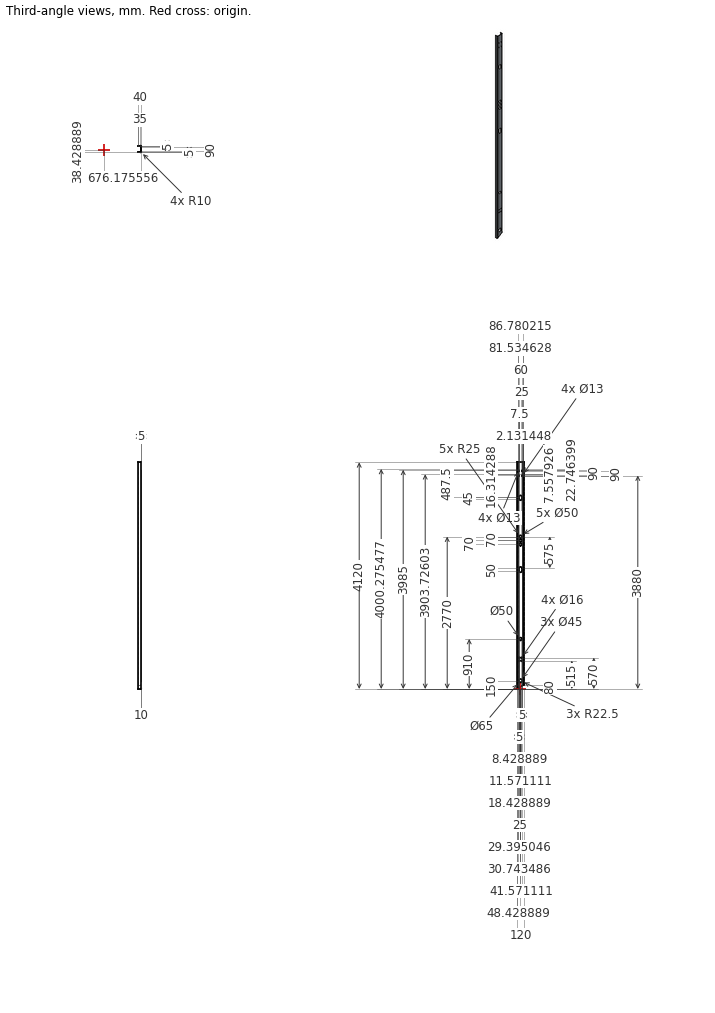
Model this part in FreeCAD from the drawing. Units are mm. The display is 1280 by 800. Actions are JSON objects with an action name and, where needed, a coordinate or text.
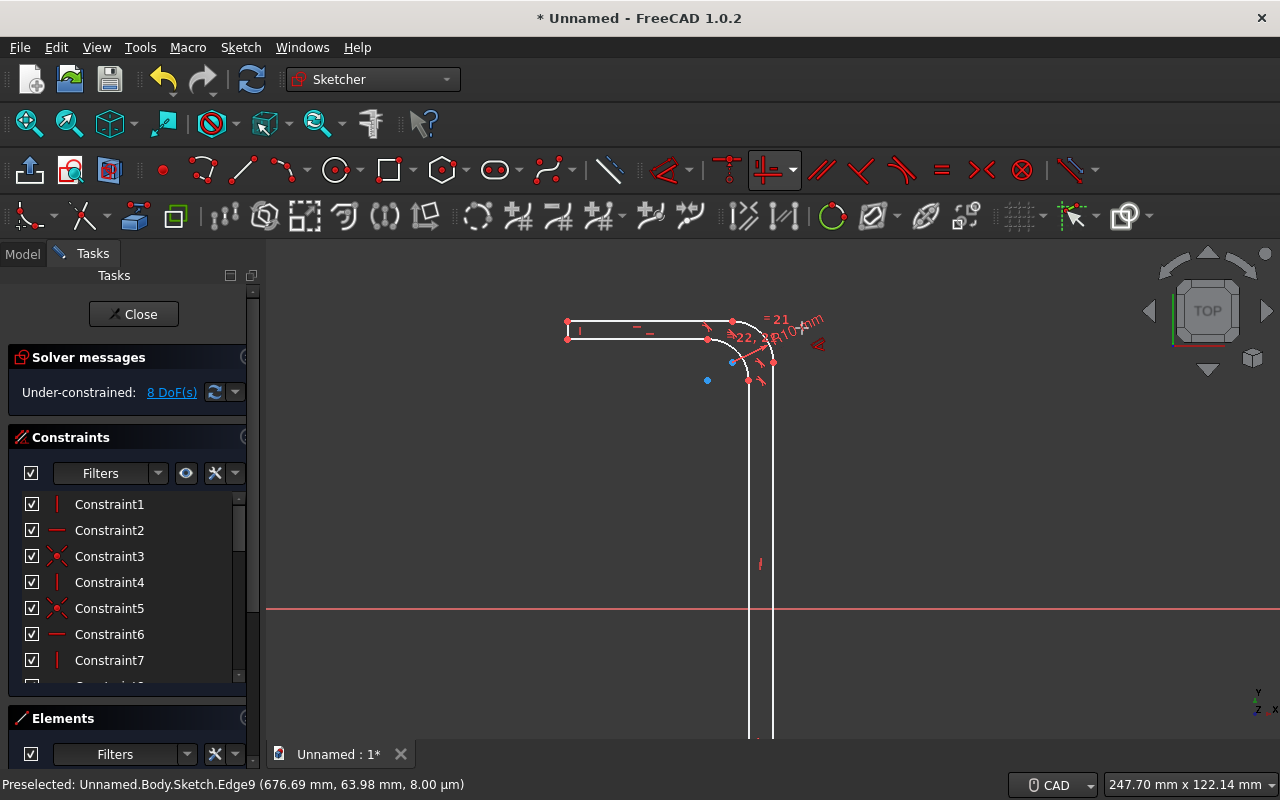
{"action": "scroll", "coordinate": [568, 330], "scroll_direction": "up", "scroll_amount": 4}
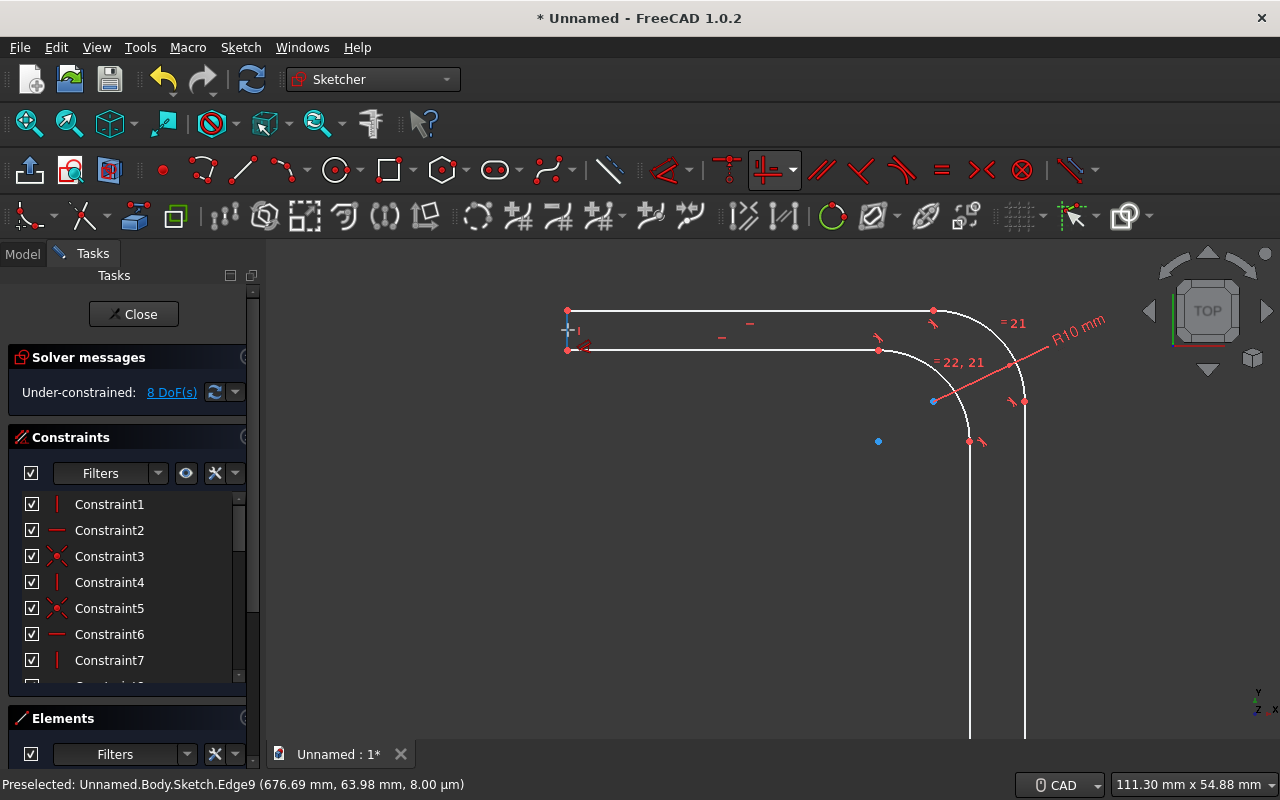
{"action": "left_click", "coordinate": [567, 330]}
{"action": "left_click", "coordinate": [533, 330]}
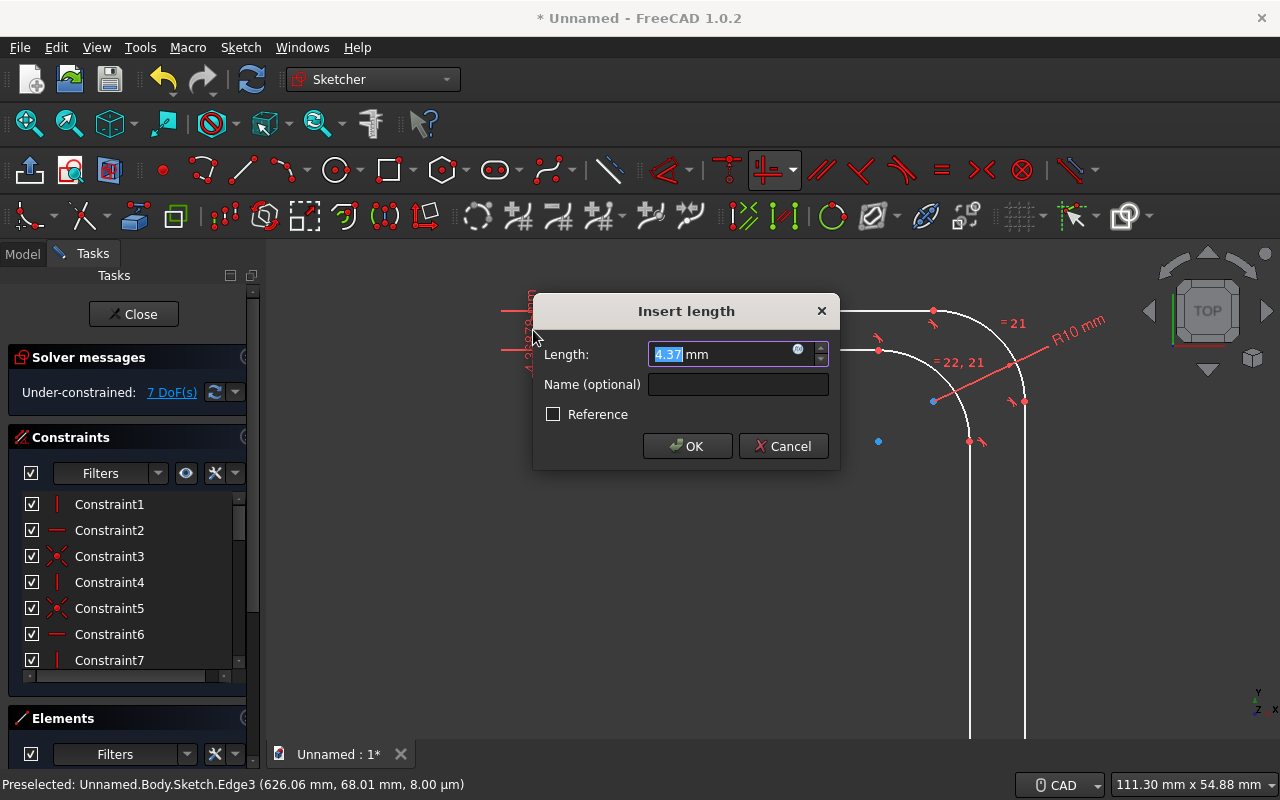
{"action": "type", "text": "5"}
{"action": "key", "text": "Return"}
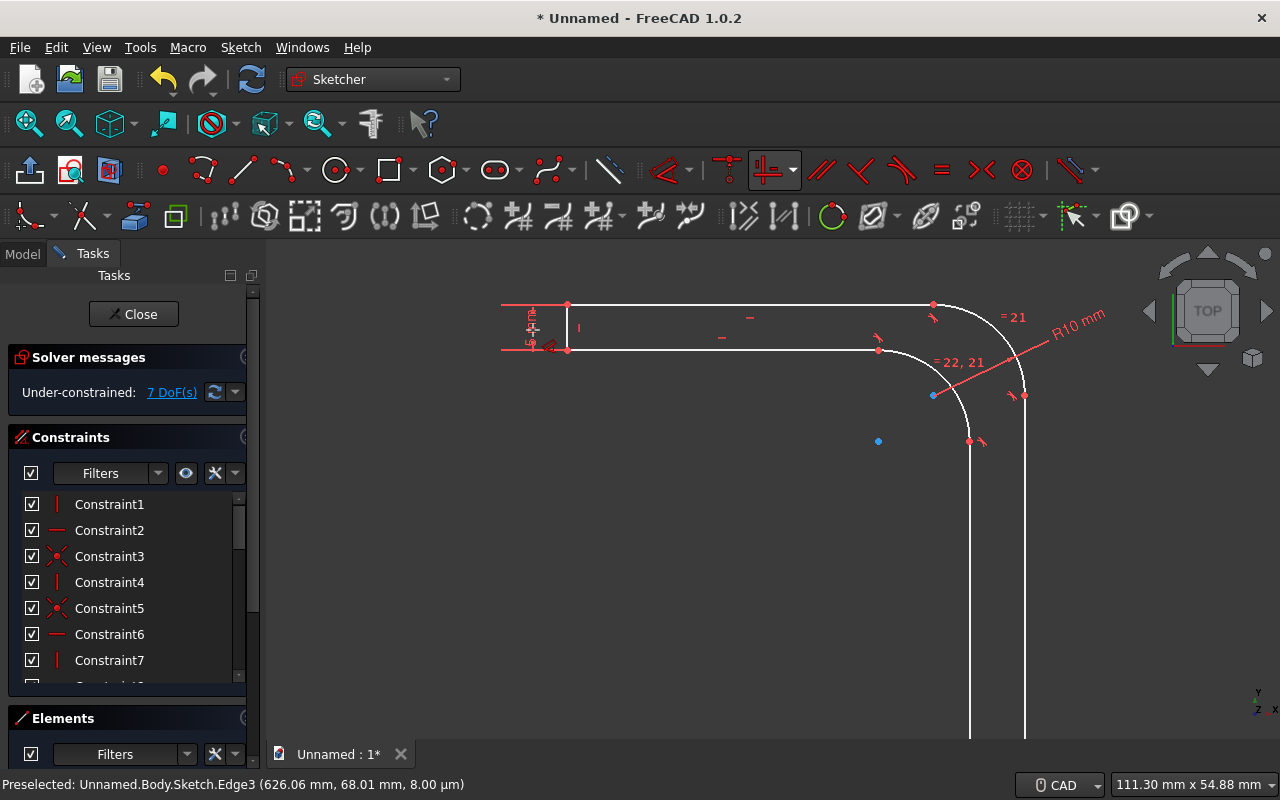
{"action": "scroll", "coordinate": [665, 335], "scroll_direction": "down", "scroll_amount": 6}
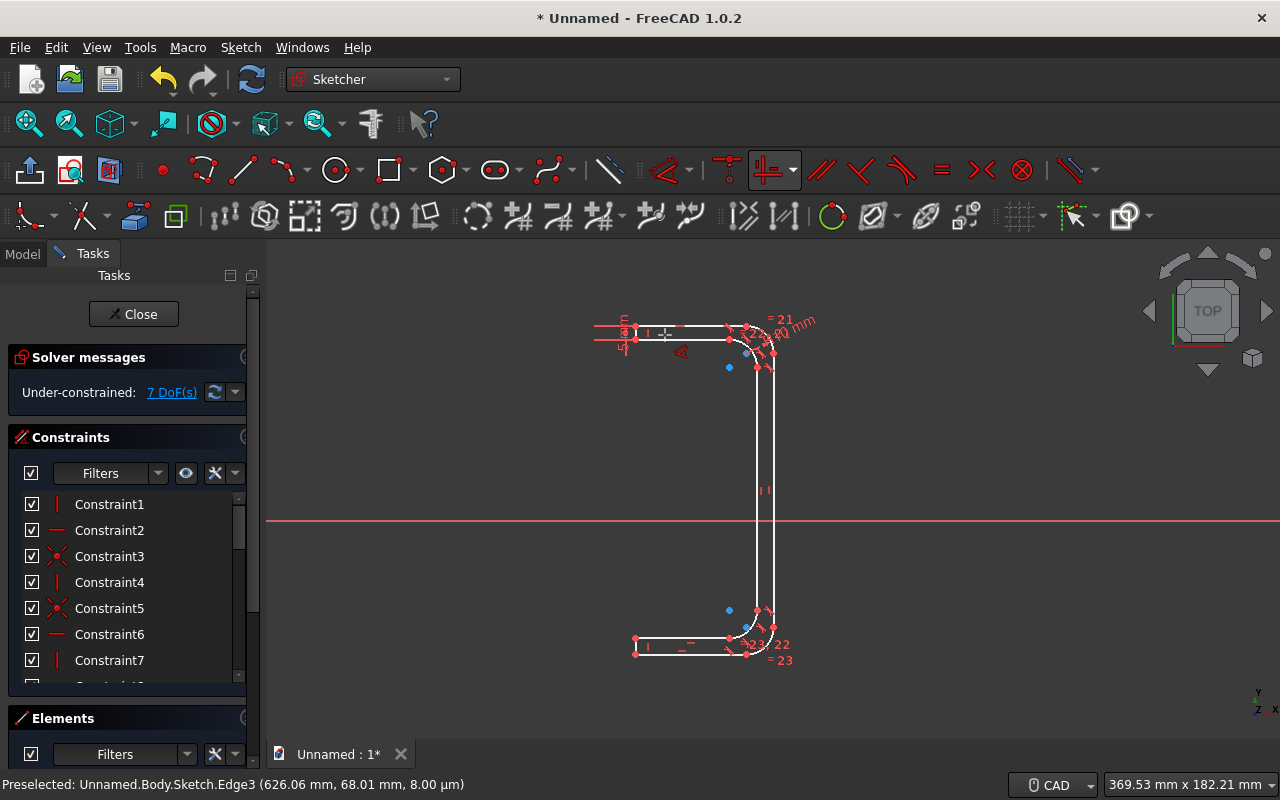
{"action": "scroll", "coordinate": [636, 643], "scroll_direction": "up", "scroll_amount": 6}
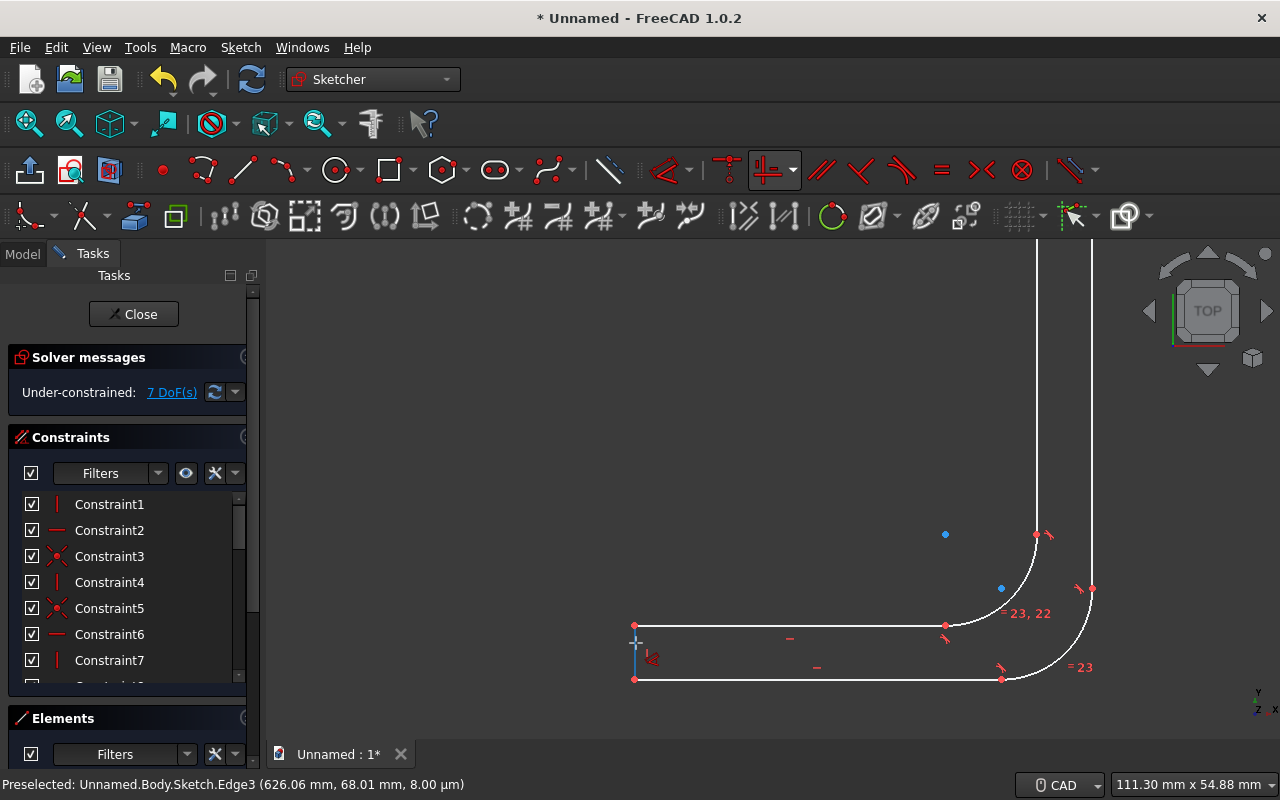
{"action": "left_click", "coordinate": [635, 642]}
{"action": "left_click", "coordinate": [601, 653]}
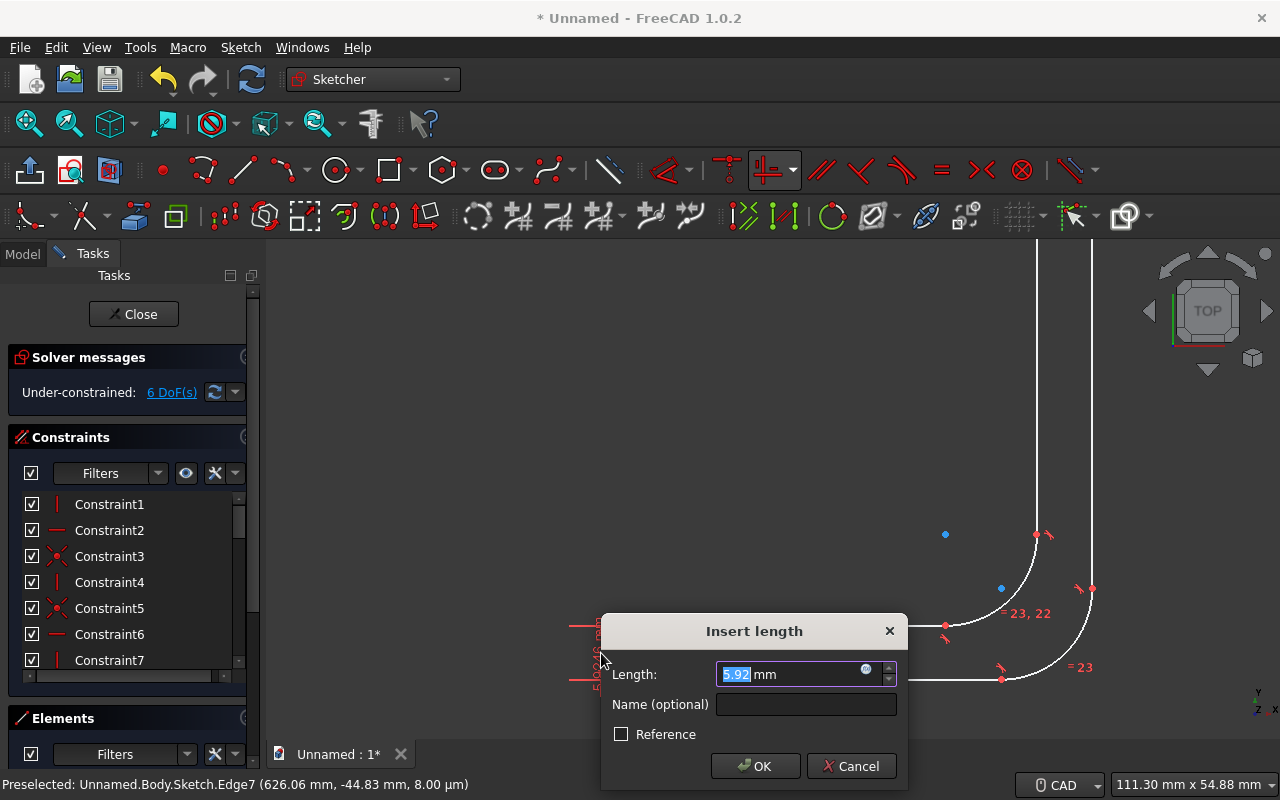
{"action": "type", "text": "5"}
{"action": "key", "text": "Return"}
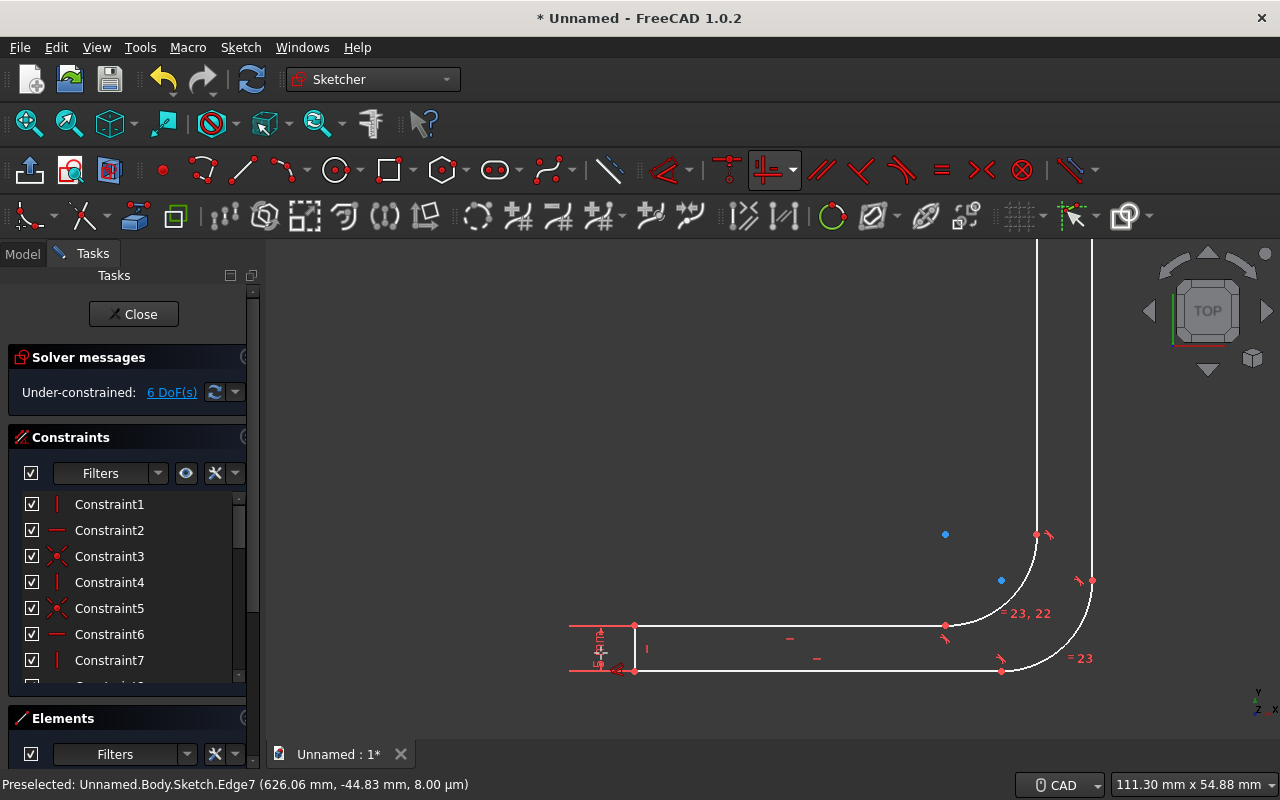
{"action": "scroll", "coordinate": [636, 644], "scroll_direction": "down", "scroll_amount": 6}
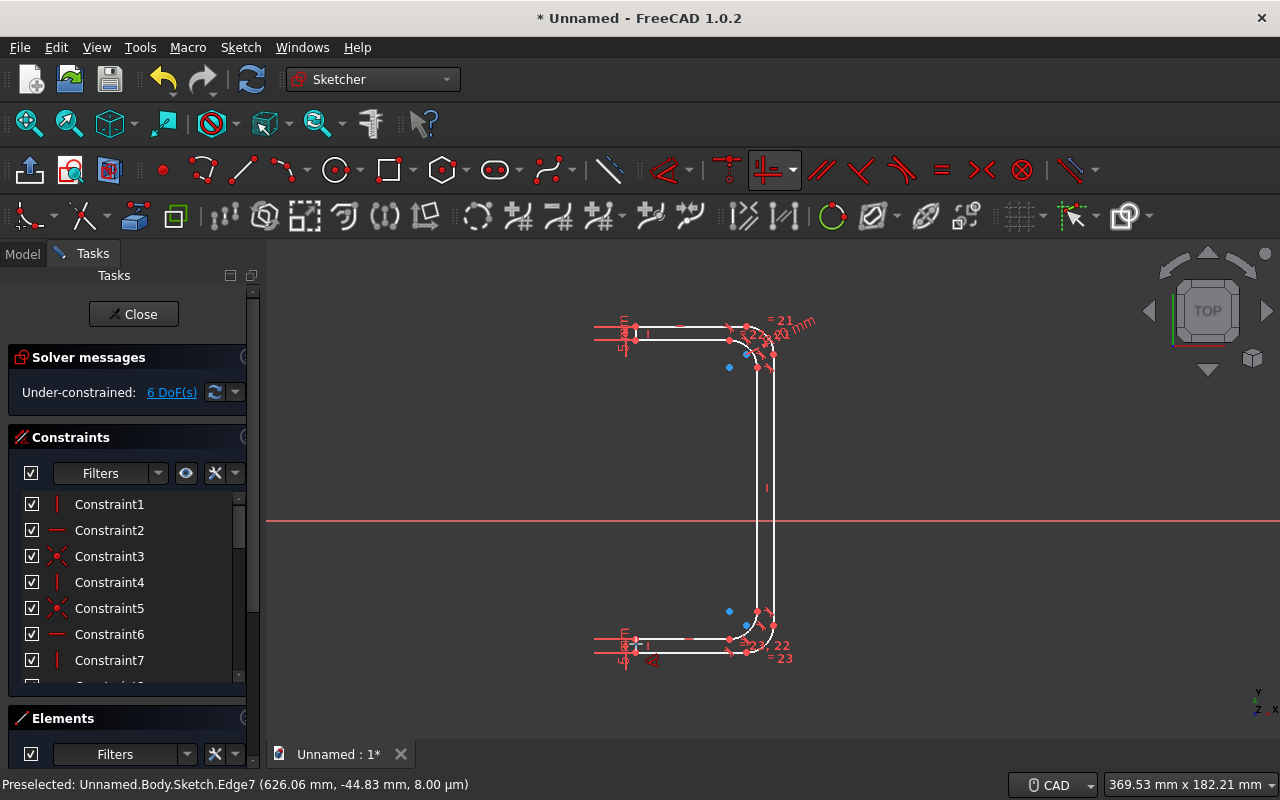
{"action": "left_click", "coordinate": [713, 327]}
{"action": "left_click", "coordinate": [691, 293]}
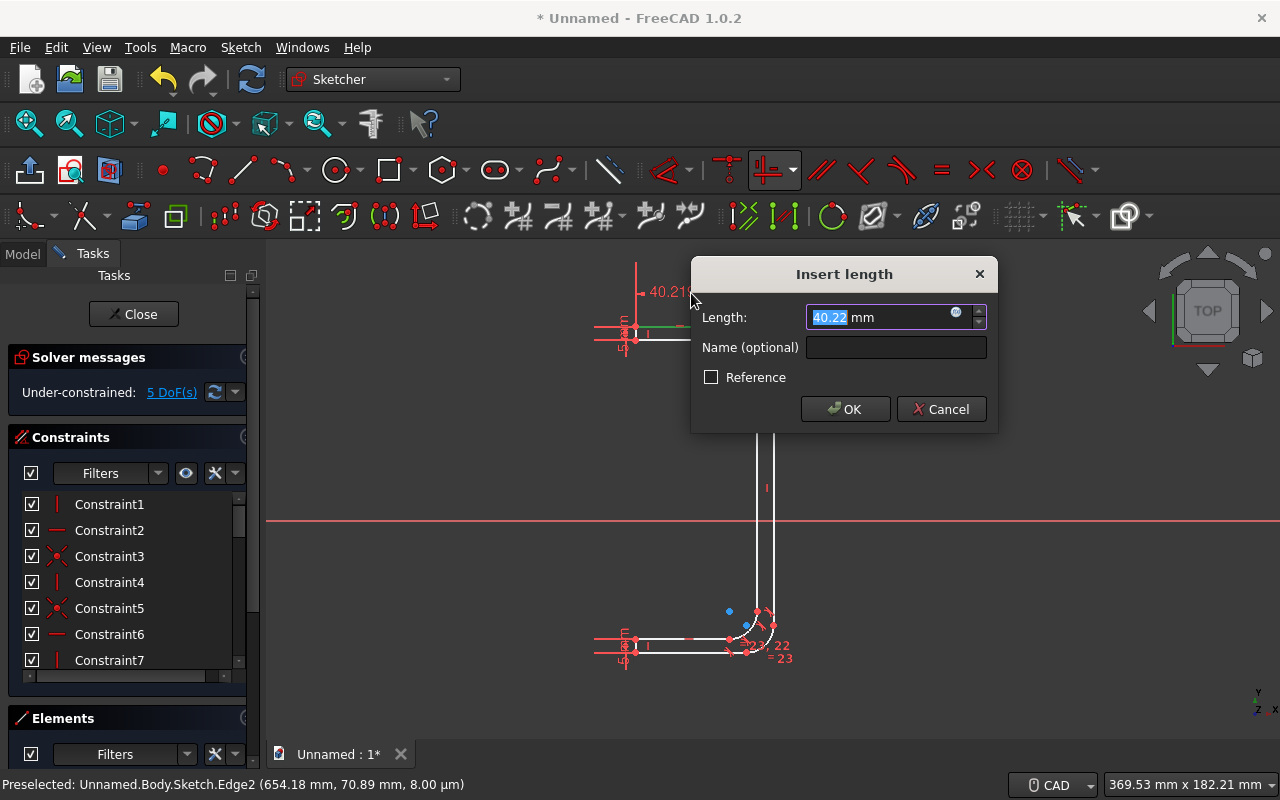
{"action": "type", "text": "40"}
{"action": "key", "text": "Return"}